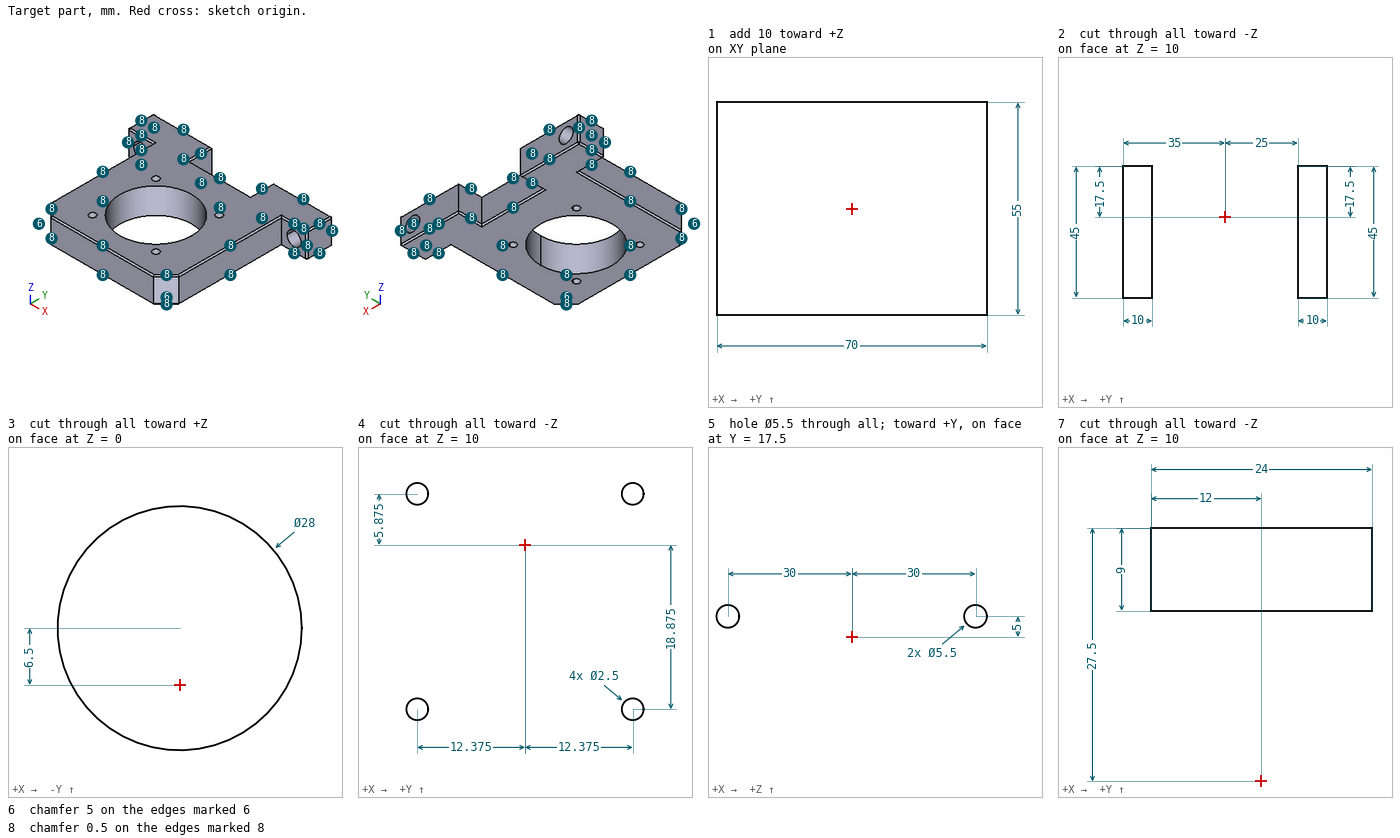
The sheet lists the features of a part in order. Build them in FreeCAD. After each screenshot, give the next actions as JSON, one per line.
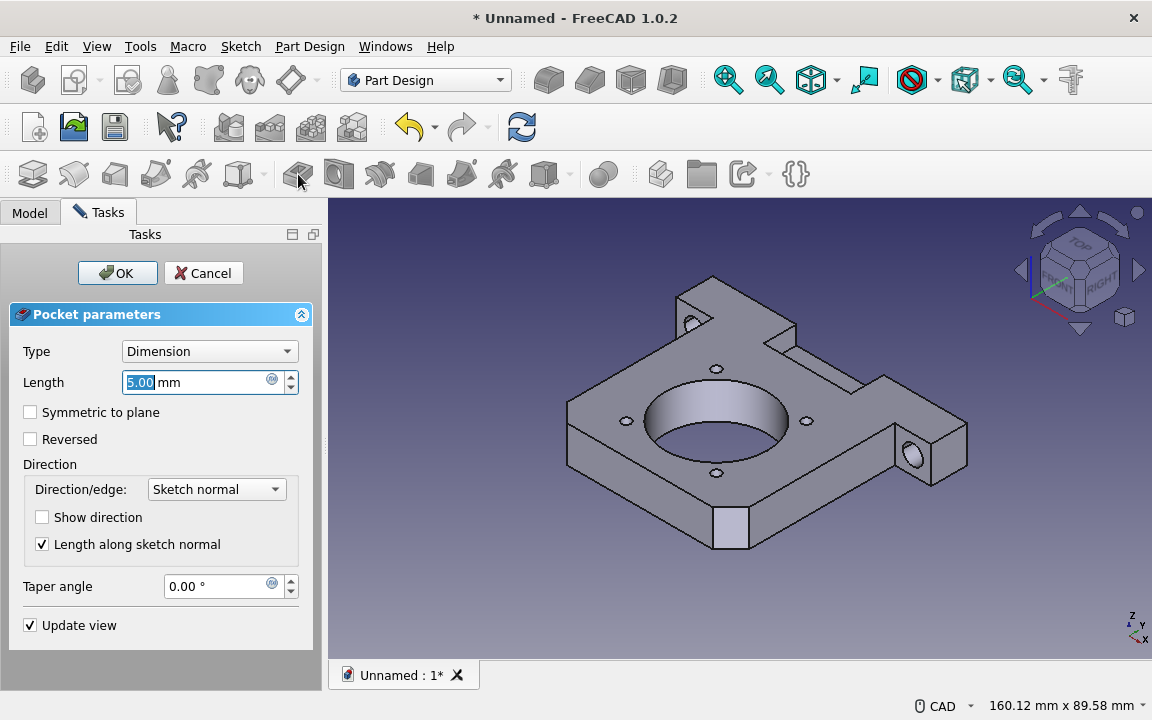
{"action": "left_click", "coordinate": [210, 352]}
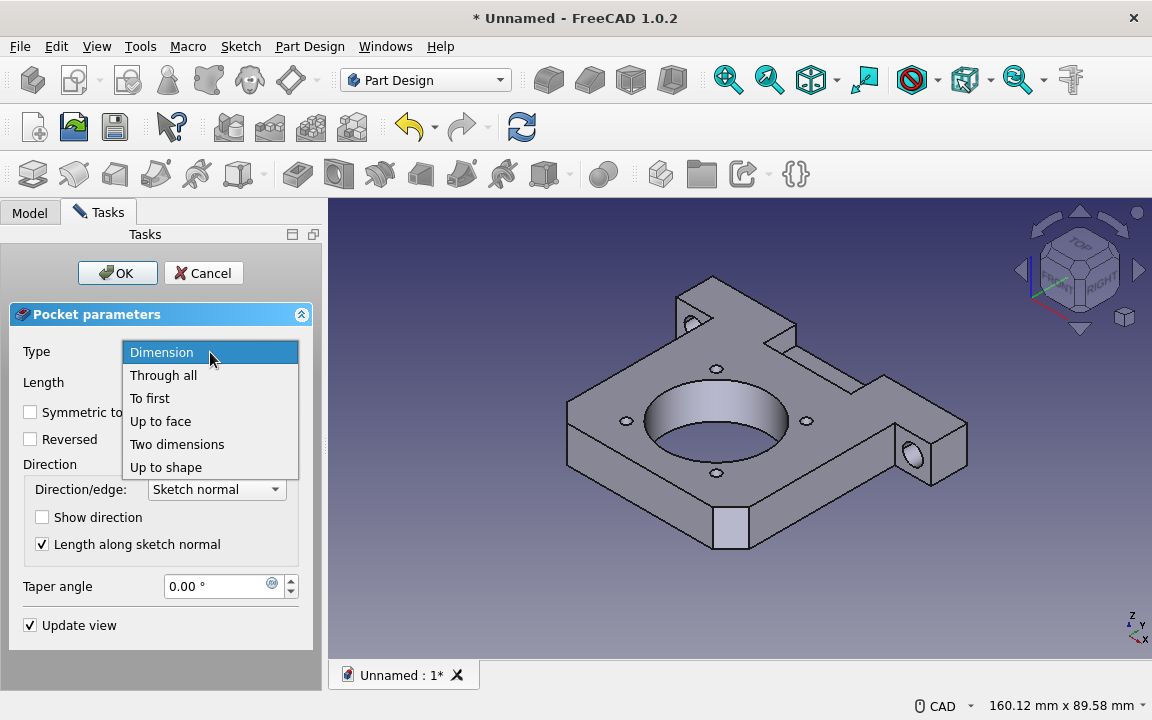
{"action": "left_click", "coordinate": [208, 376]}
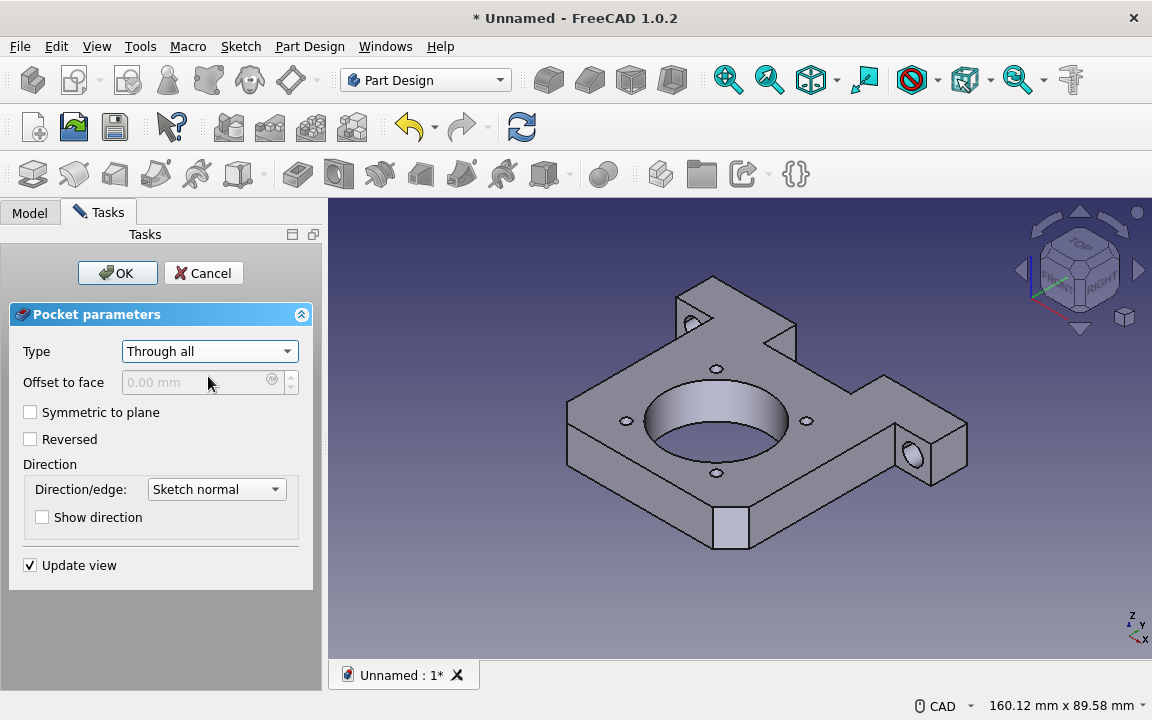
{"action": "left_click", "coordinate": [118, 273]}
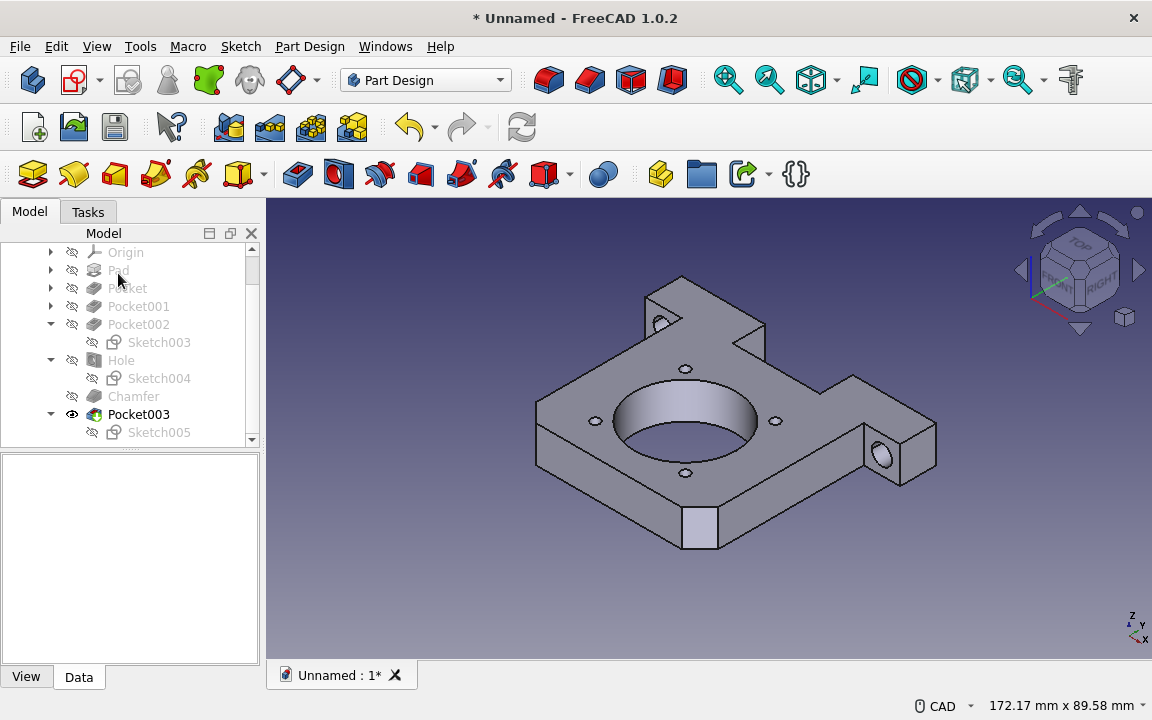
{"action": "left_click", "coordinate": [918, 454]}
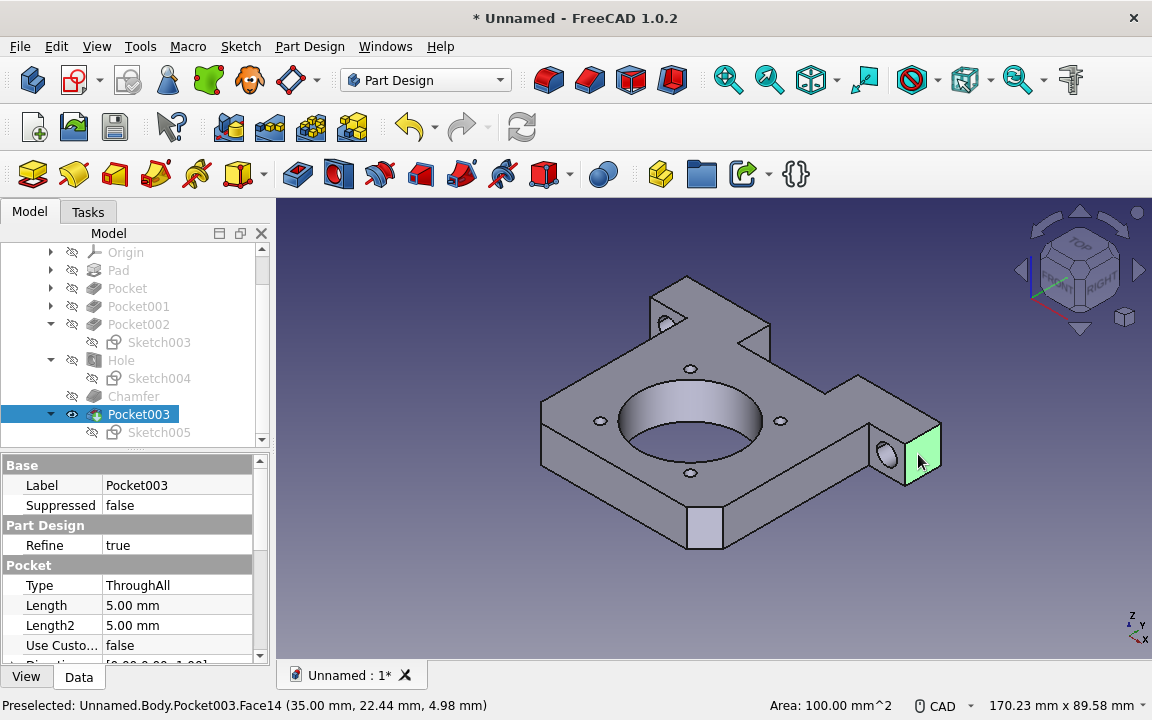
{"action": "left_click", "coordinate": [669, 307], "text": "ctrl"}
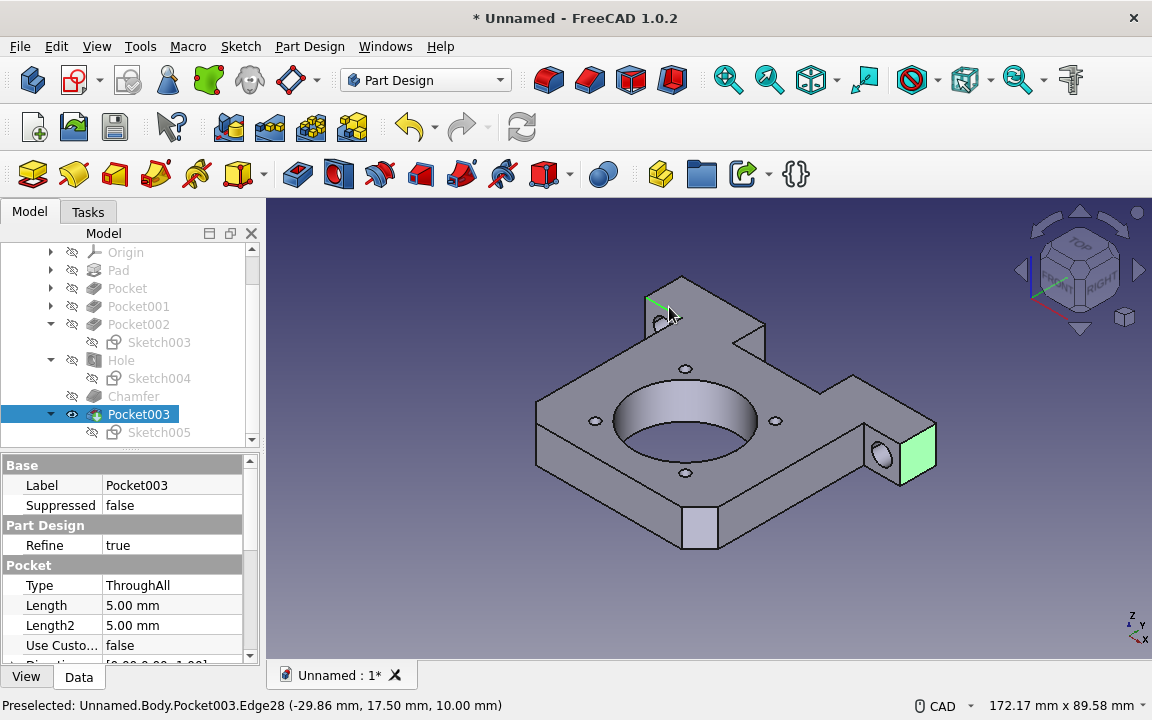
{"action": "left_click", "coordinate": [882, 433], "text": "ctrl"}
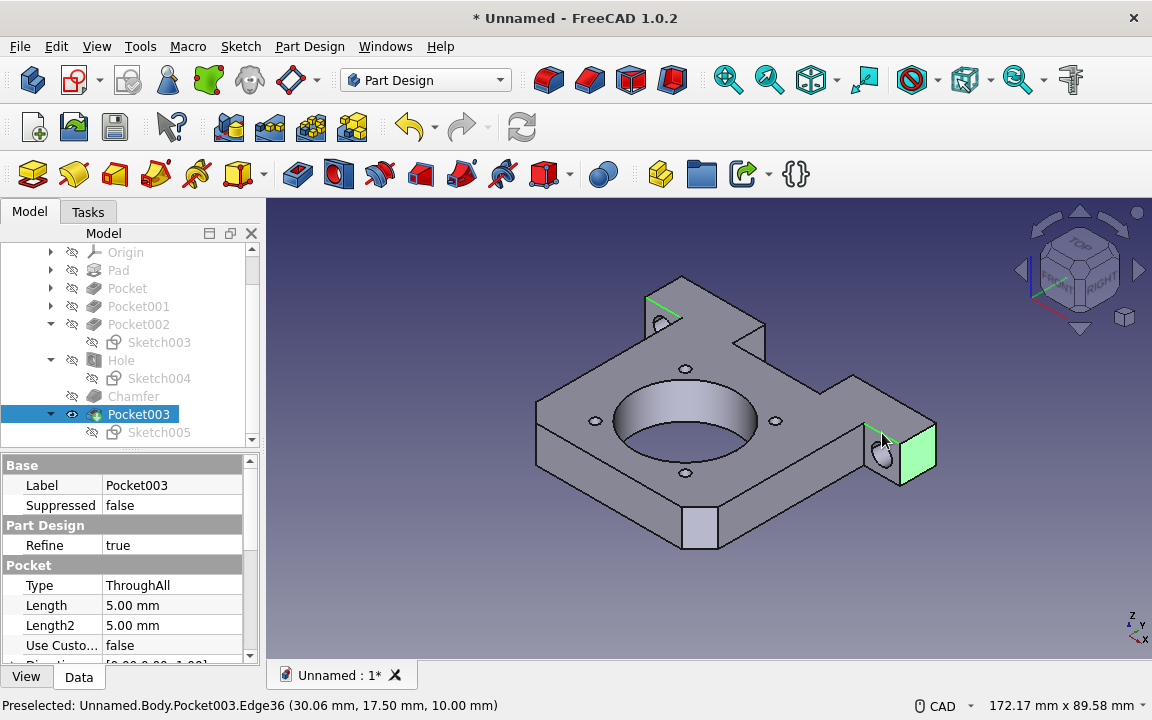
{"action": "left_click", "coordinate": [791, 464], "text": "ctrl"}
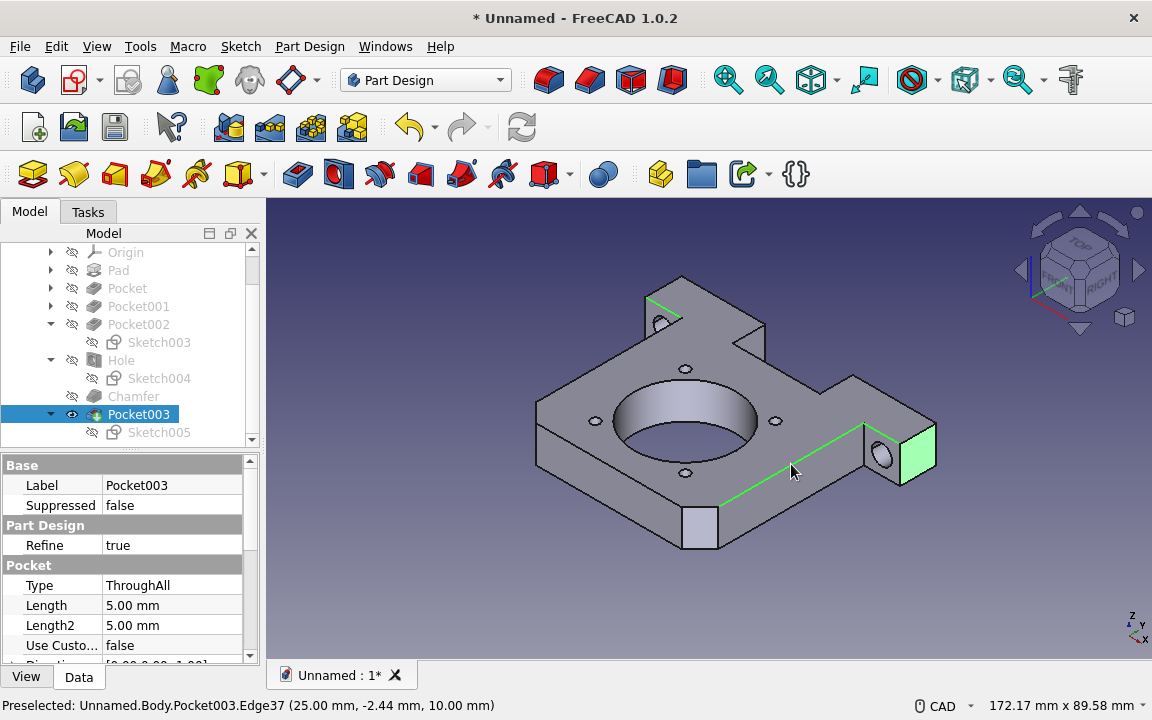
{"action": "left_click", "coordinate": [609, 464], "text": "ctrl"}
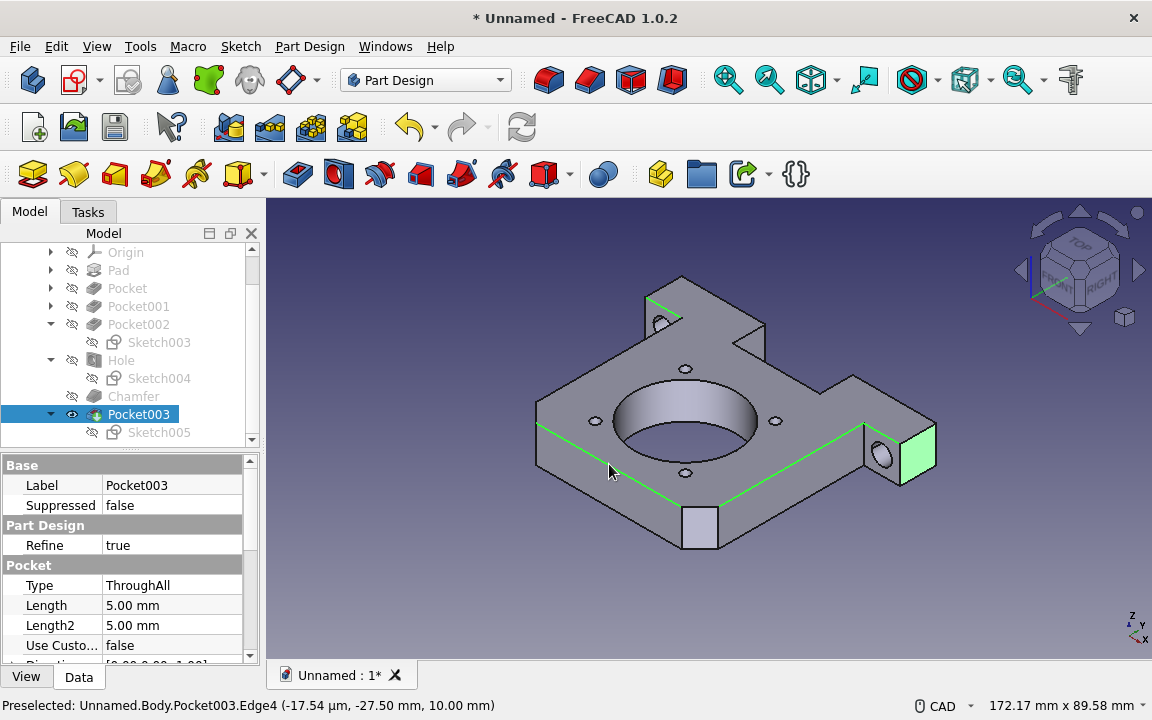
{"action": "left_click", "coordinate": [700, 506], "text": "ctrl"}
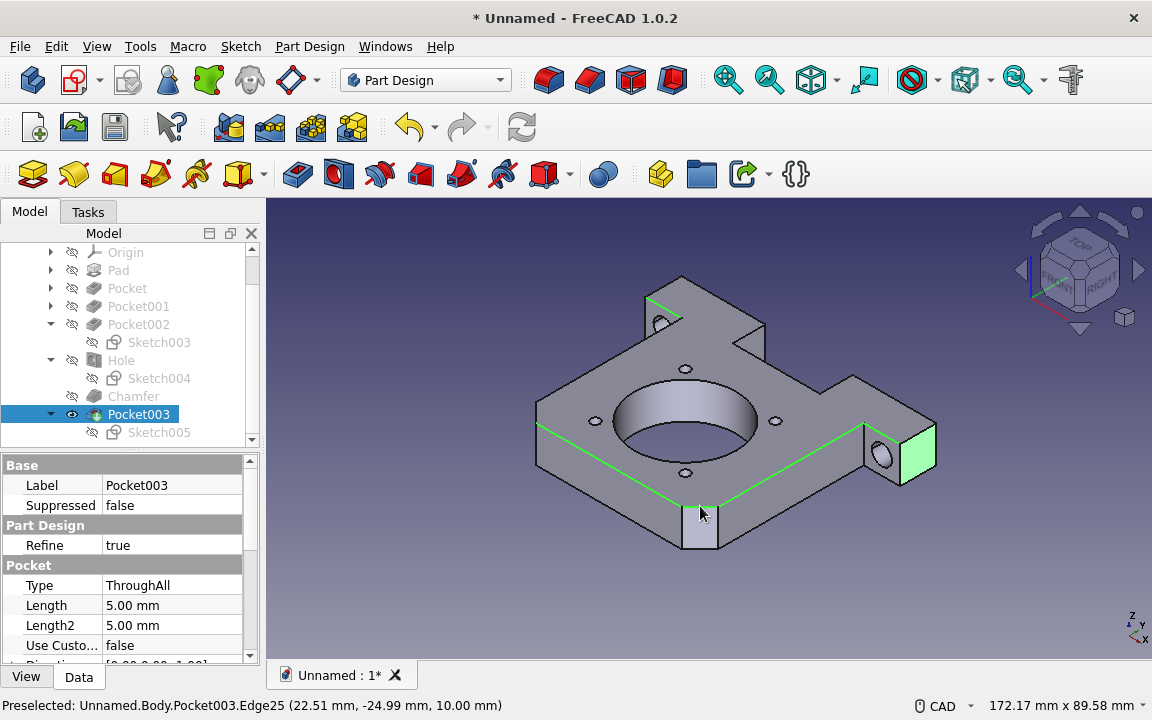
{"action": "left_click", "coordinate": [749, 333], "text": "ctrl"}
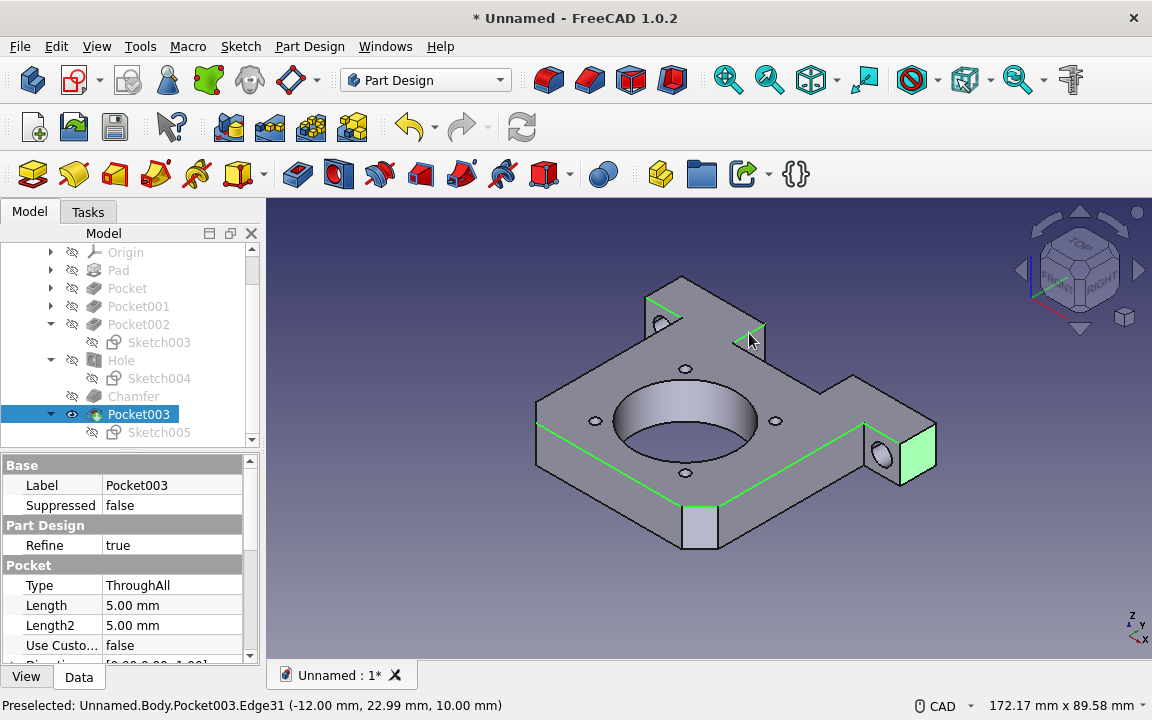
{"action": "key", "text": "2"}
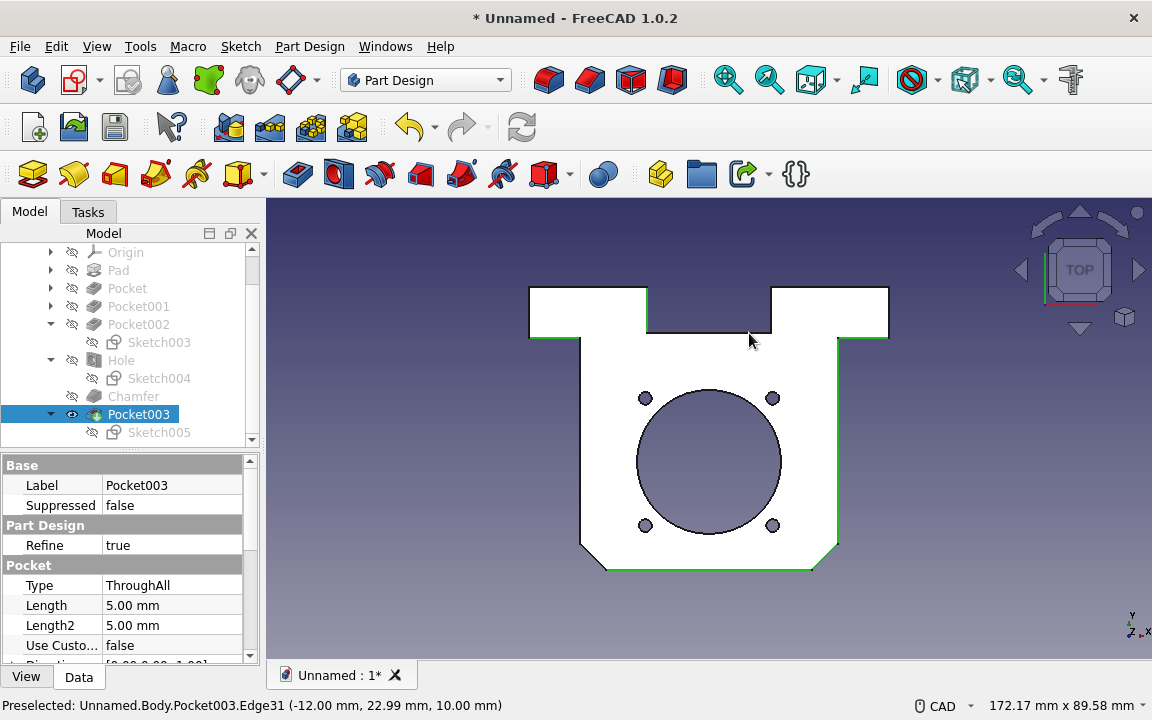
{"action": "left_click", "coordinate": [709, 332], "text": "ctrl"}